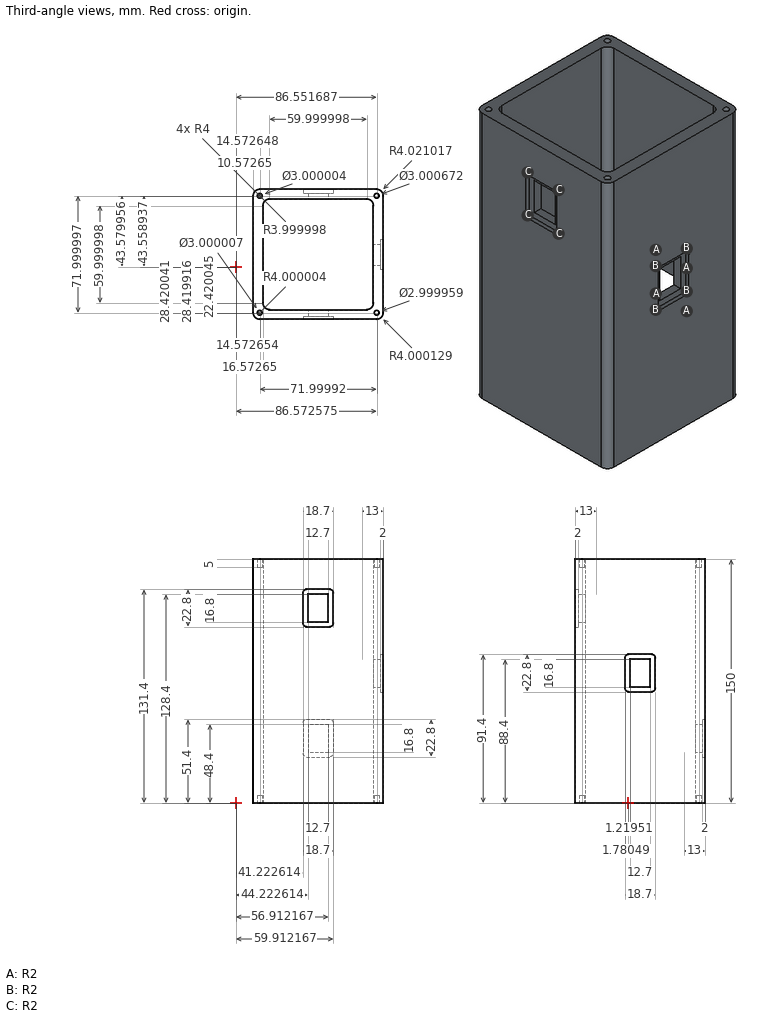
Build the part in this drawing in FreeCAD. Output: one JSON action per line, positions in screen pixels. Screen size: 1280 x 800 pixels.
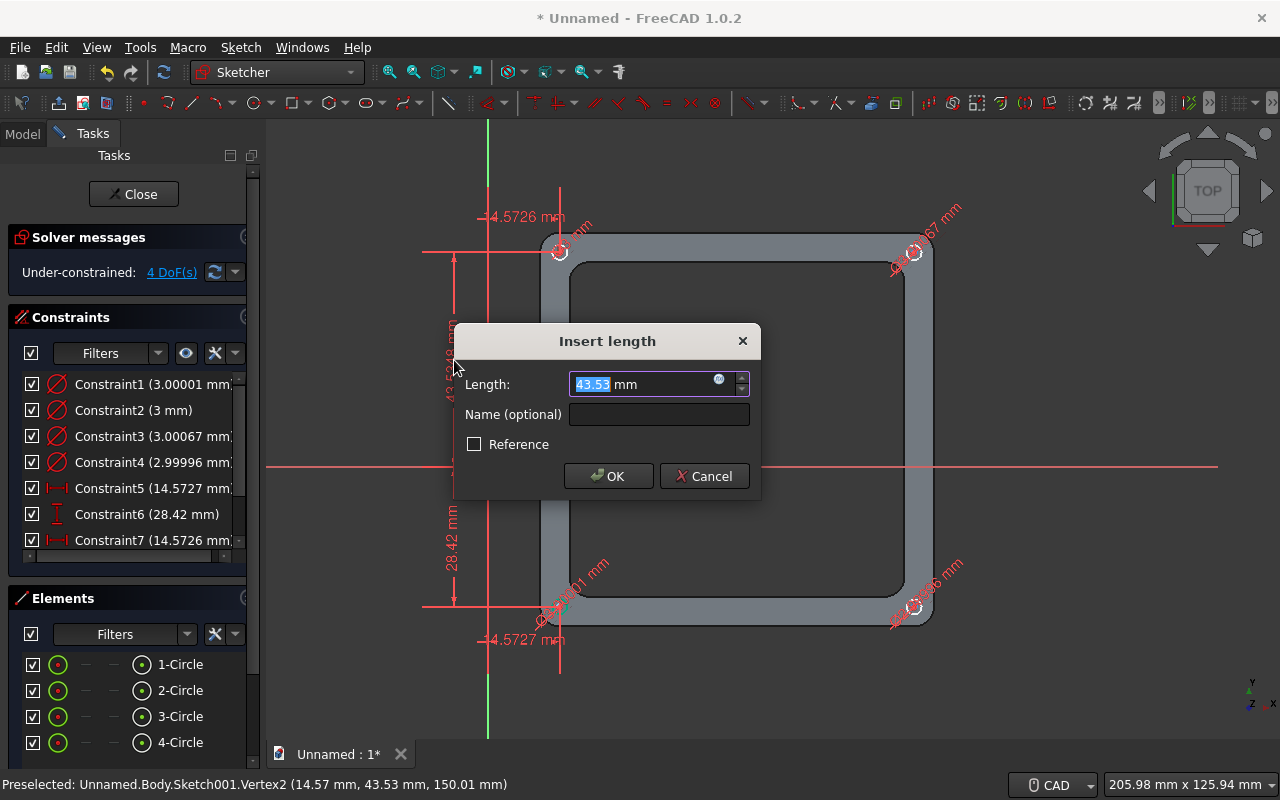
{"action": "type", "text": "43.579956"}
{"action": "key", "text": "Return"}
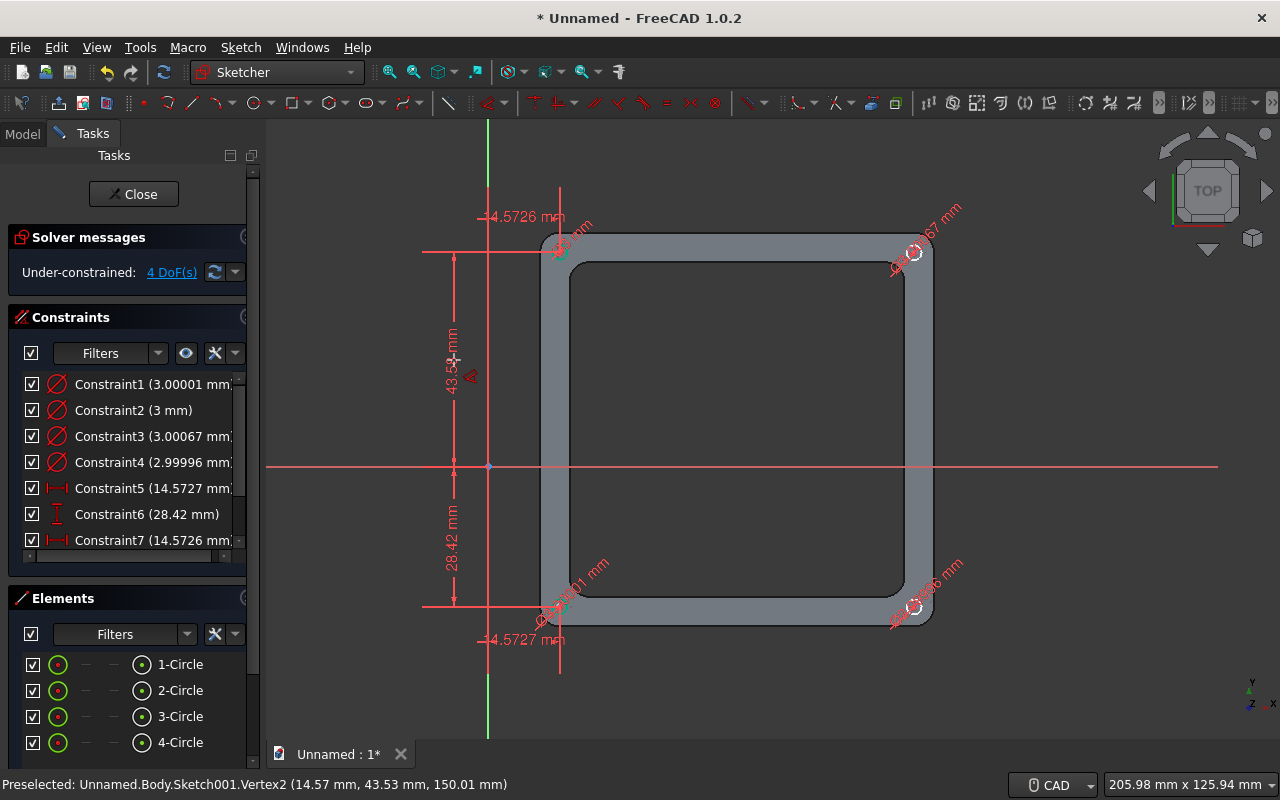
{"action": "left_click", "coordinate": [914, 253]}
{"action": "left_click", "coordinate": [701, 219]}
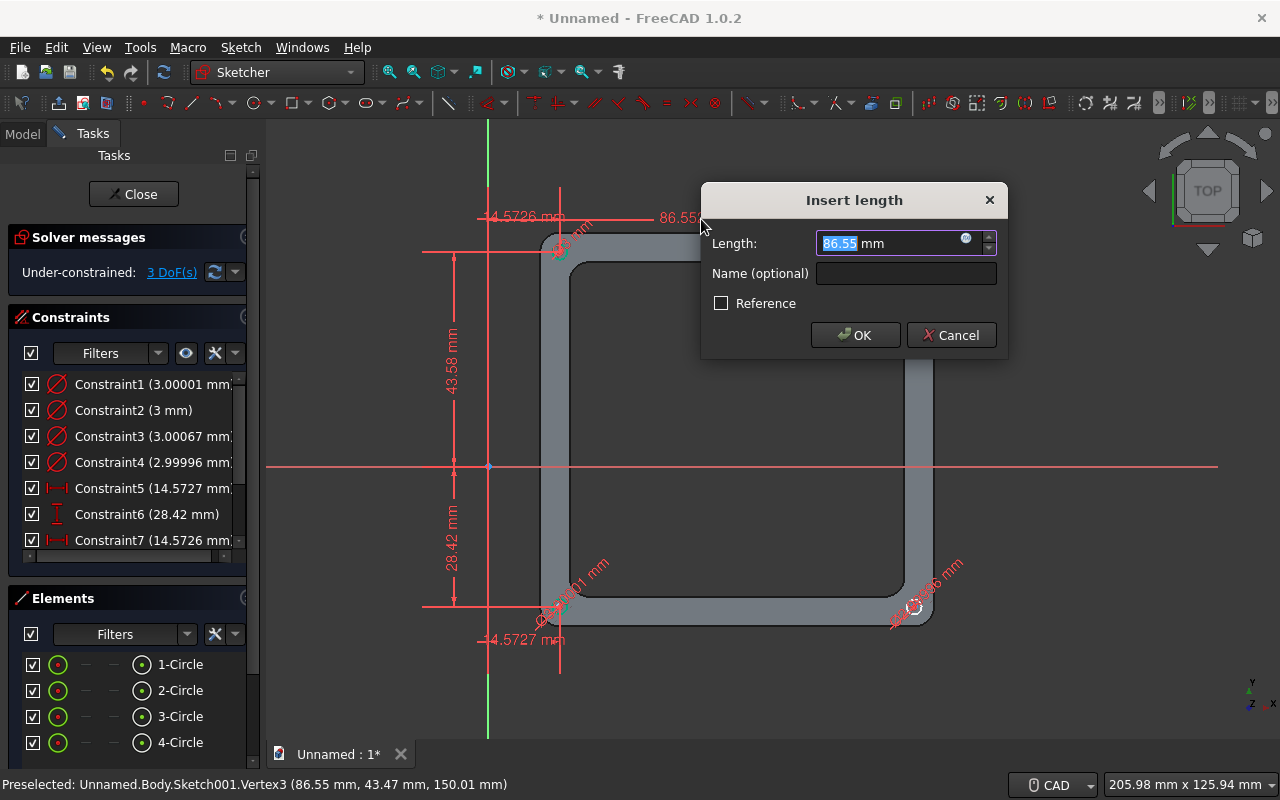
{"action": "type", "text": "86.551687"}
{"action": "key", "text": "Return"}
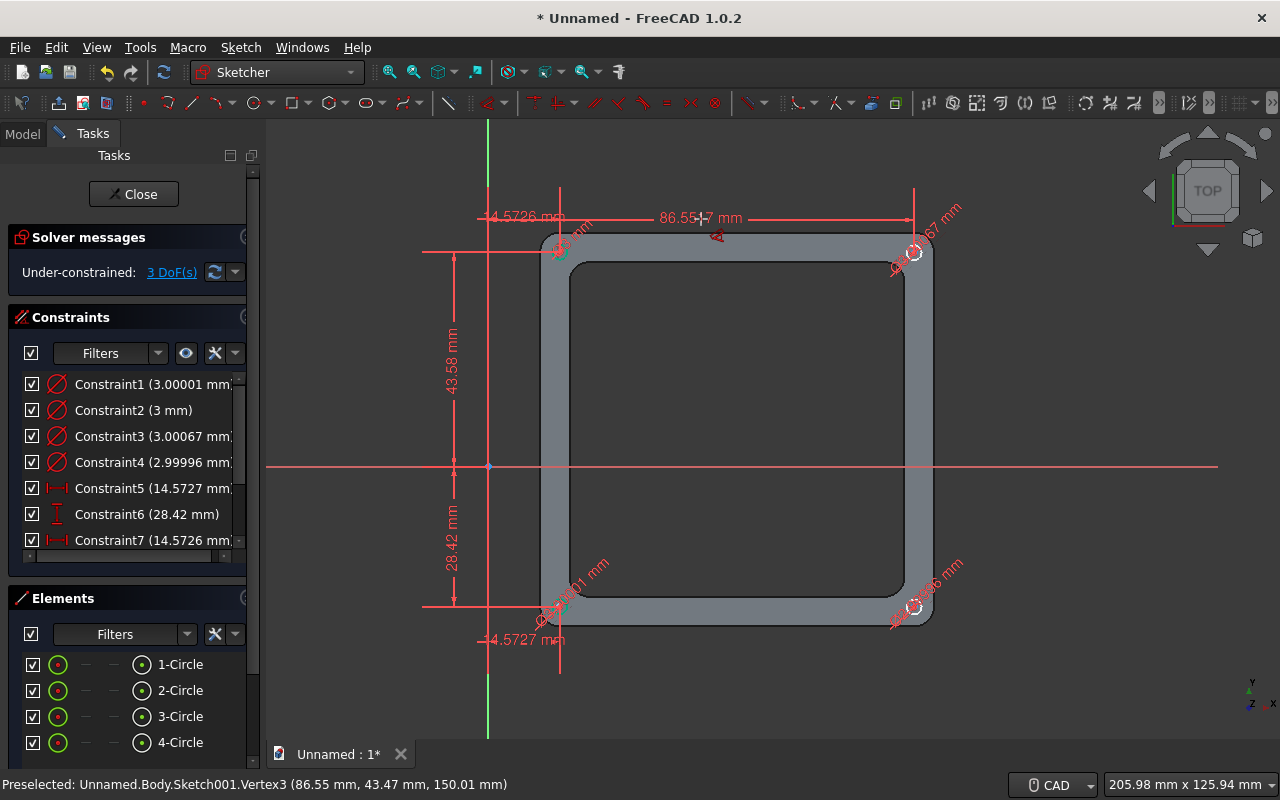
{"action": "left_click", "coordinate": [914, 253]}
{"action": "left_click", "coordinate": [454, 311]}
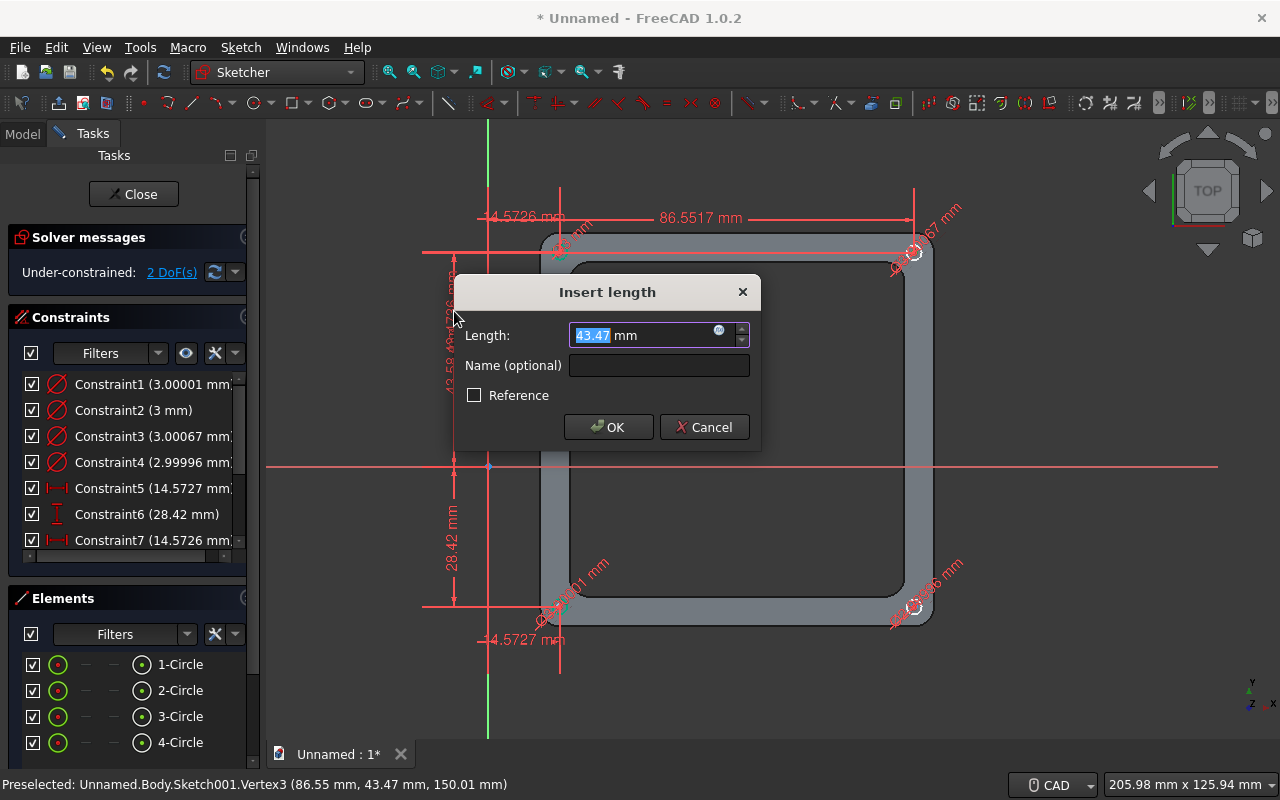
{"action": "type", "text": "43.558937"}
{"action": "key", "text": "Return"}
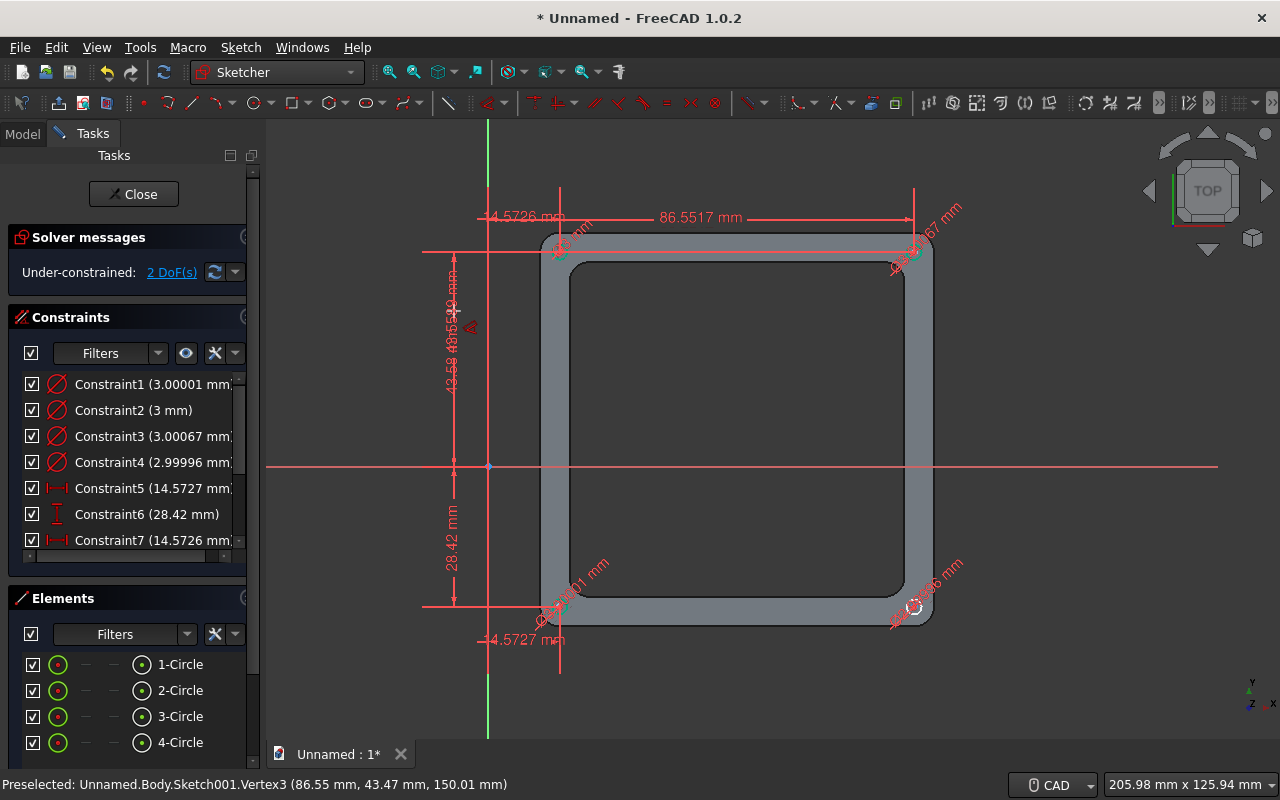
{"action": "left_click", "coordinate": [914, 607]}
{"action": "left_click", "coordinate": [701, 641]}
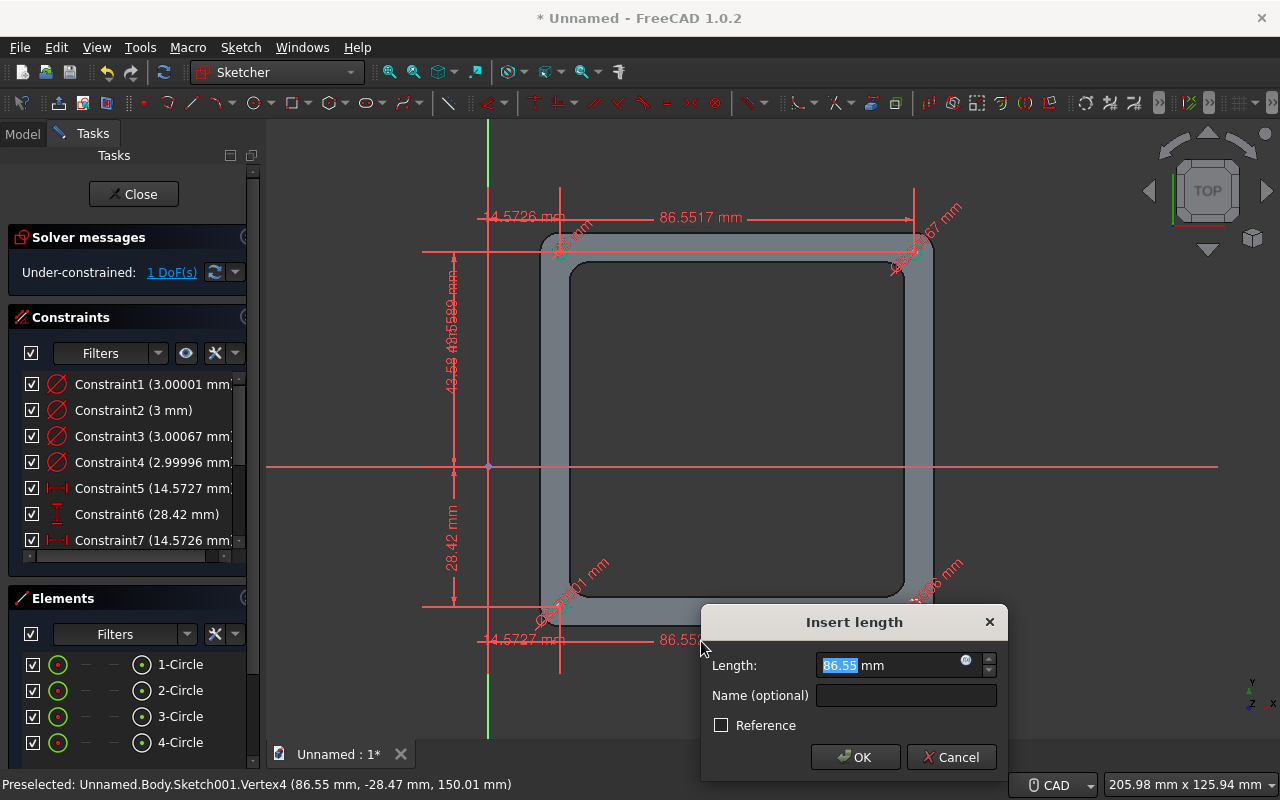
{"action": "type", "text": "86.572575"}
{"action": "key", "text": "Return"}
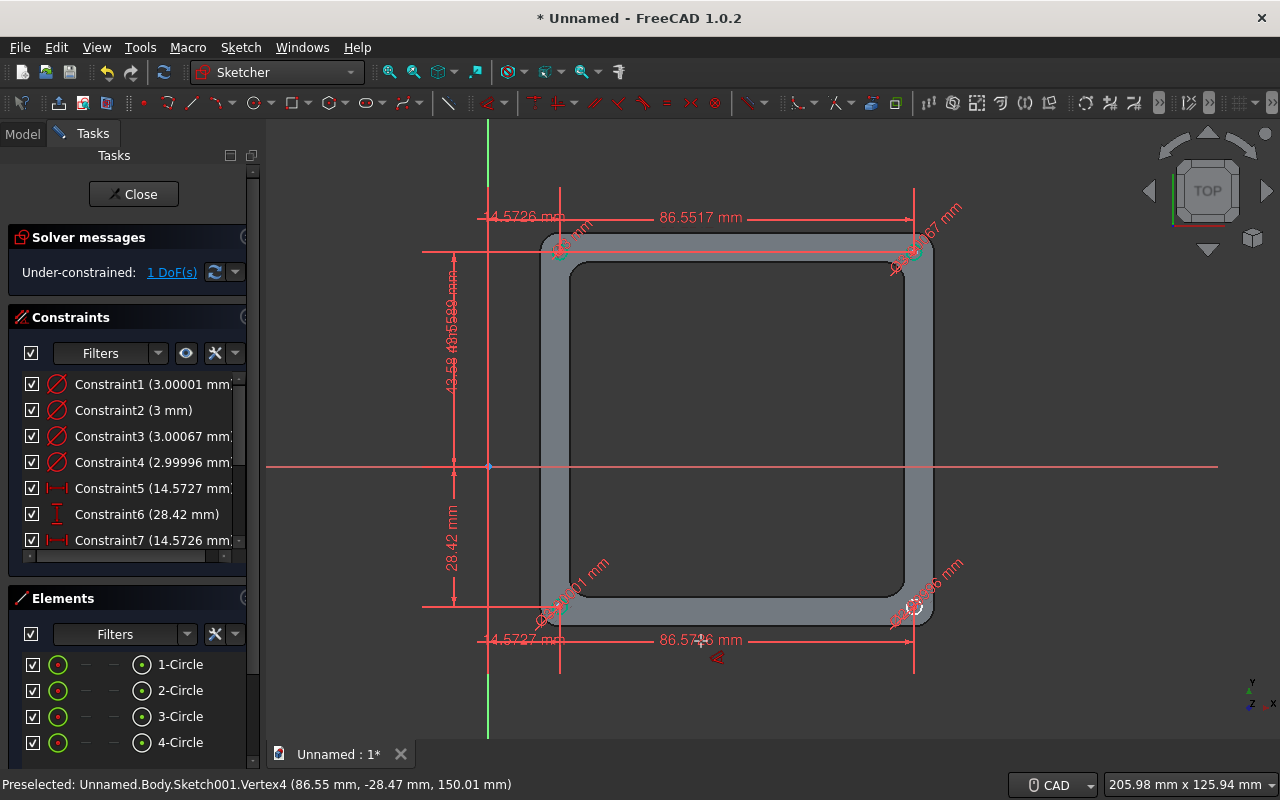
{"action": "left_click", "coordinate": [914, 607]}
{"action": "left_click", "coordinate": [454, 505]}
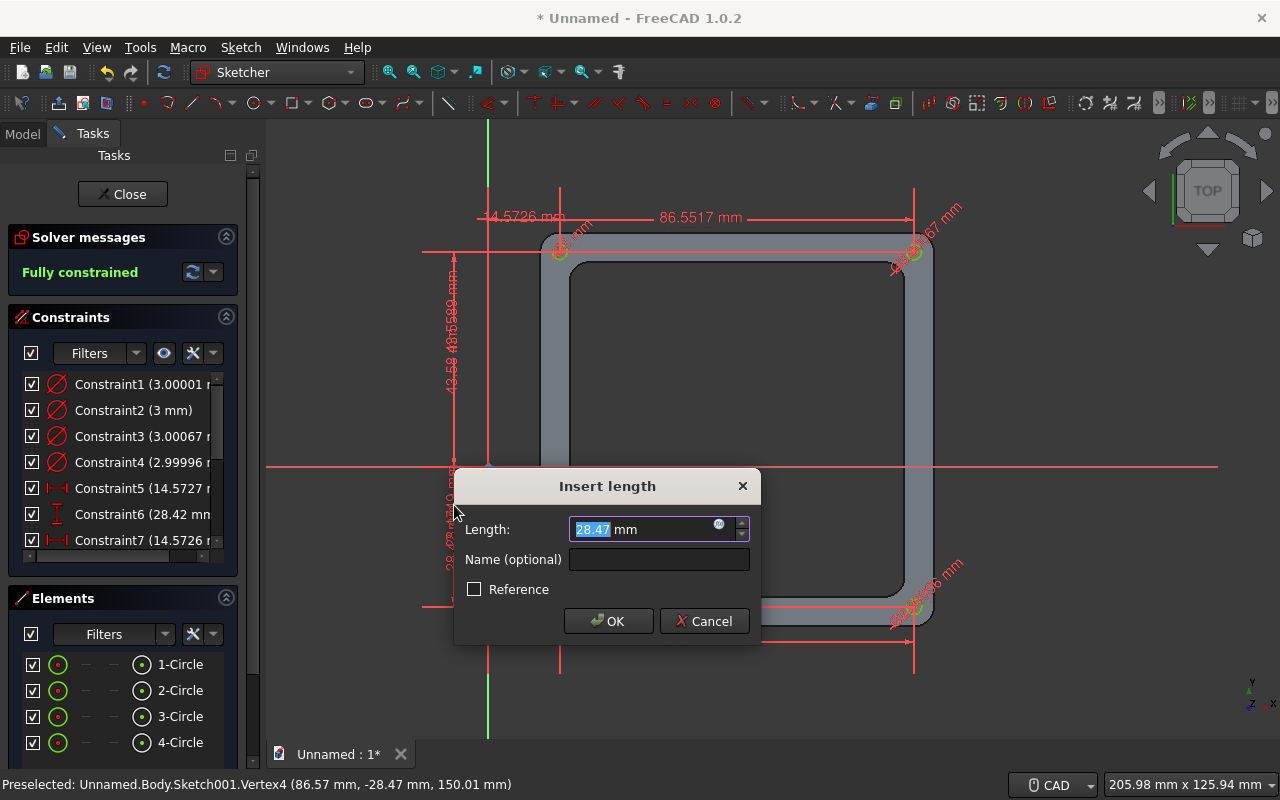
{"action": "type", "text": "28.419916"}
{"action": "key", "text": "Return"}
{"action": "key", "text": "Escape"}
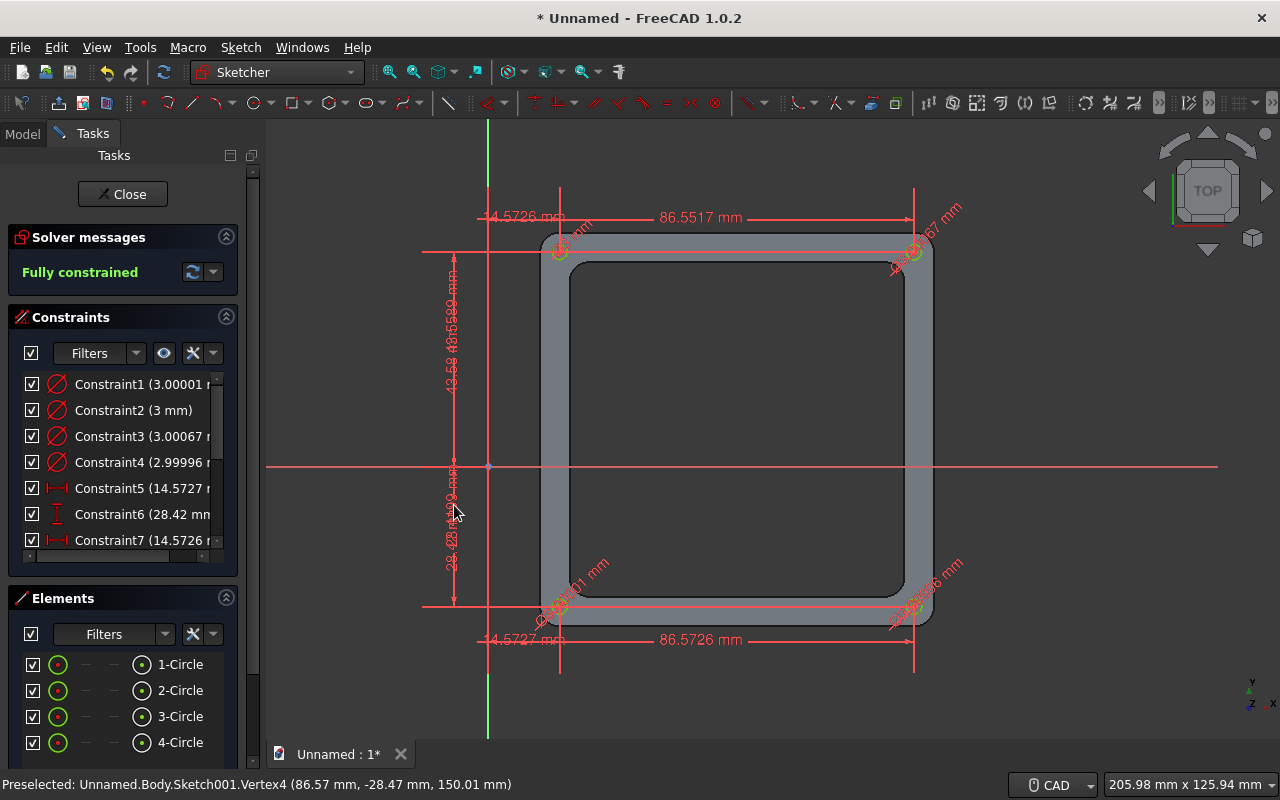
{"action": "left_click", "coordinate": [123, 194]}